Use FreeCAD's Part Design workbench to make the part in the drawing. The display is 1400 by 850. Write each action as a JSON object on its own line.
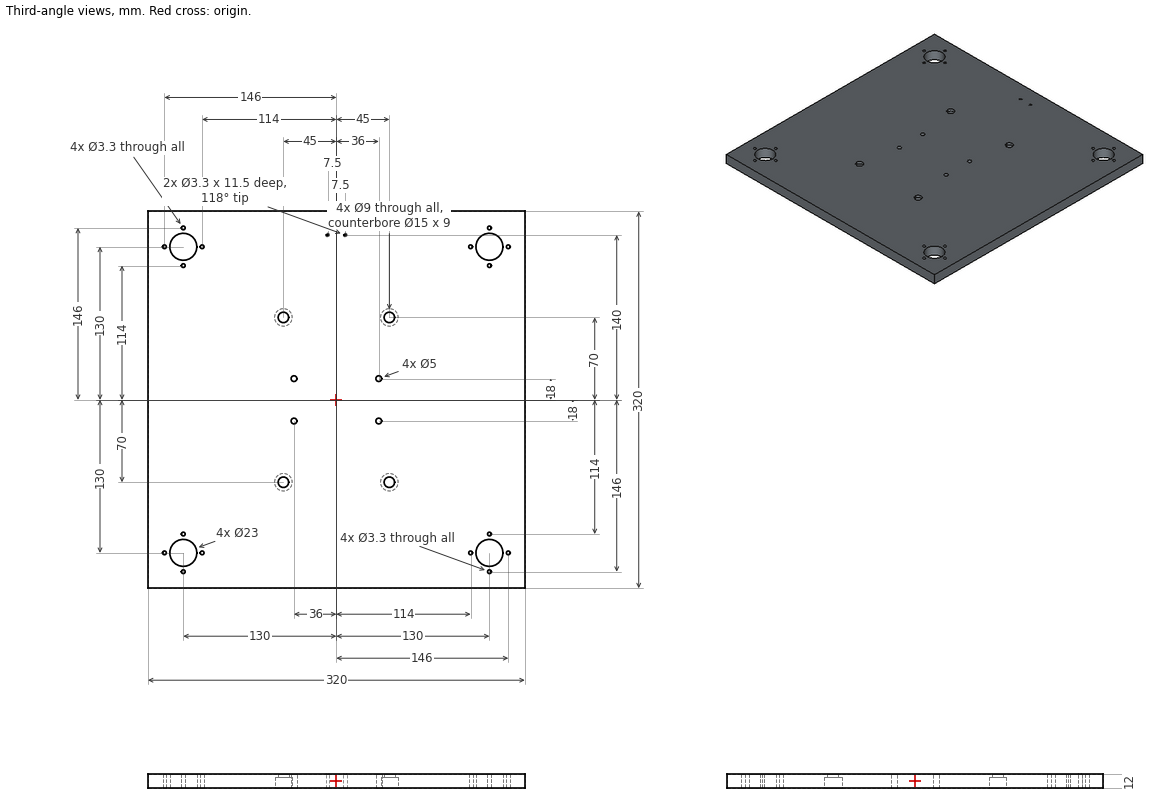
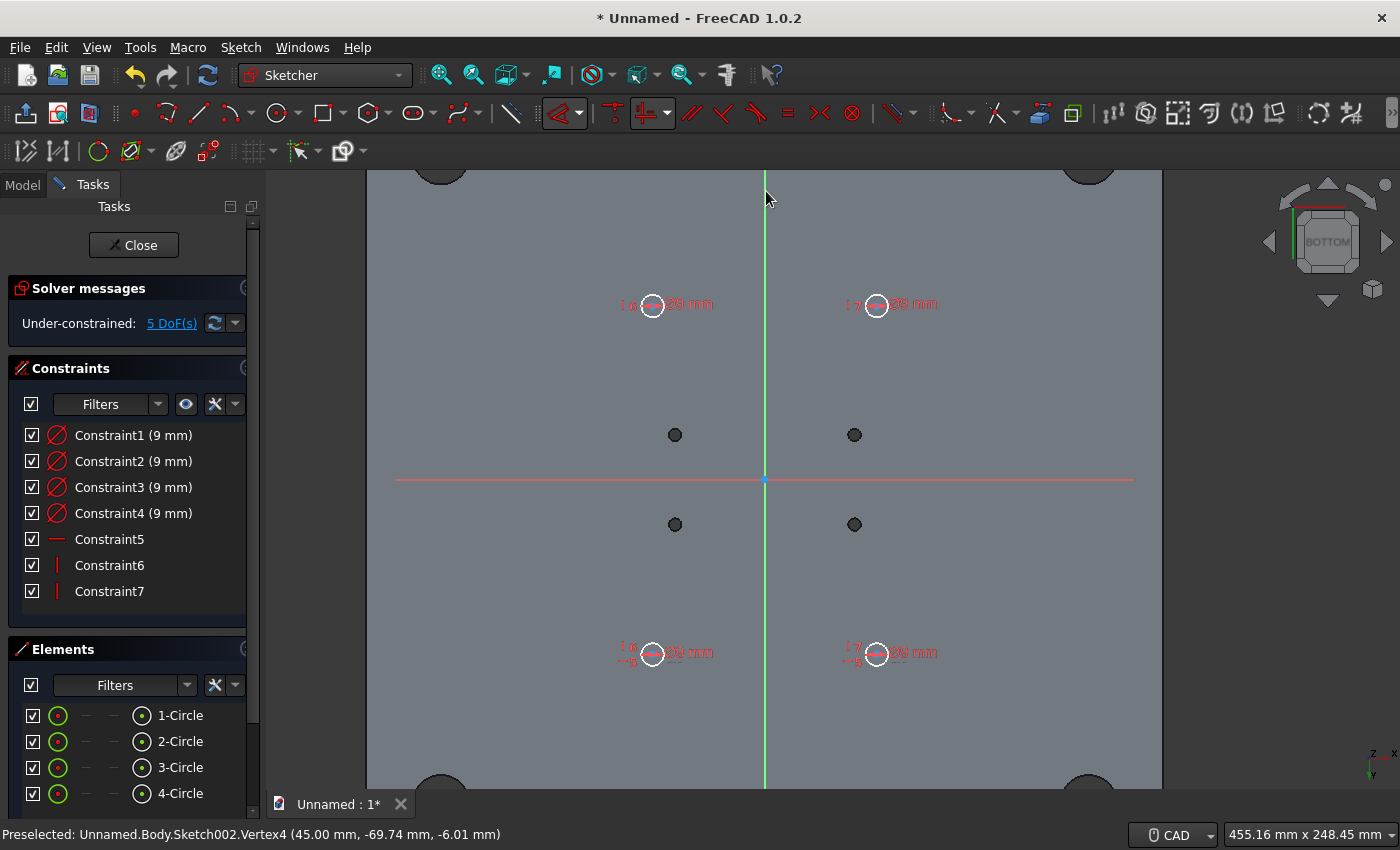
{"action": "left_click", "coordinate": [653, 306]}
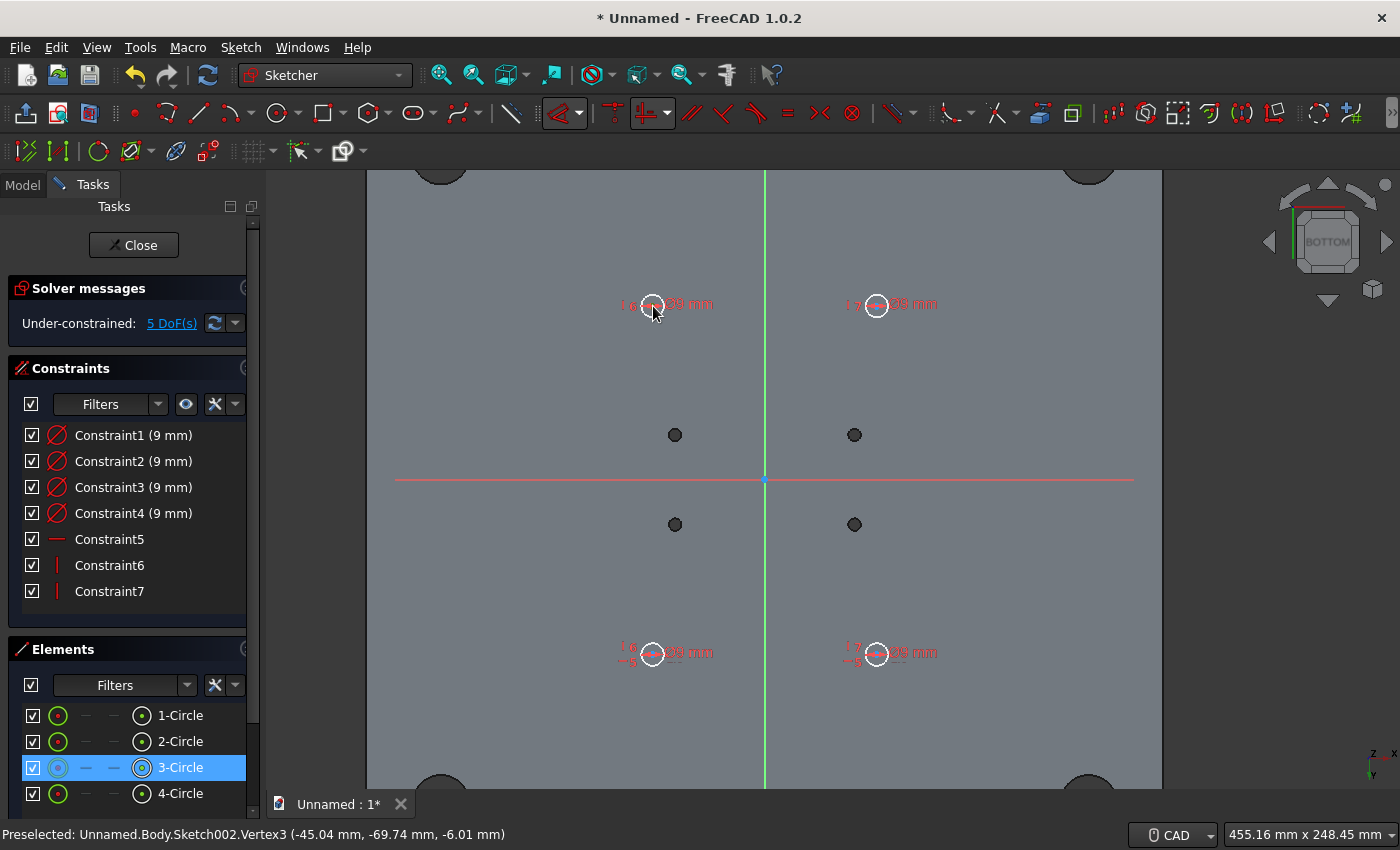
{"action": "left_click", "coordinate": [877, 306]}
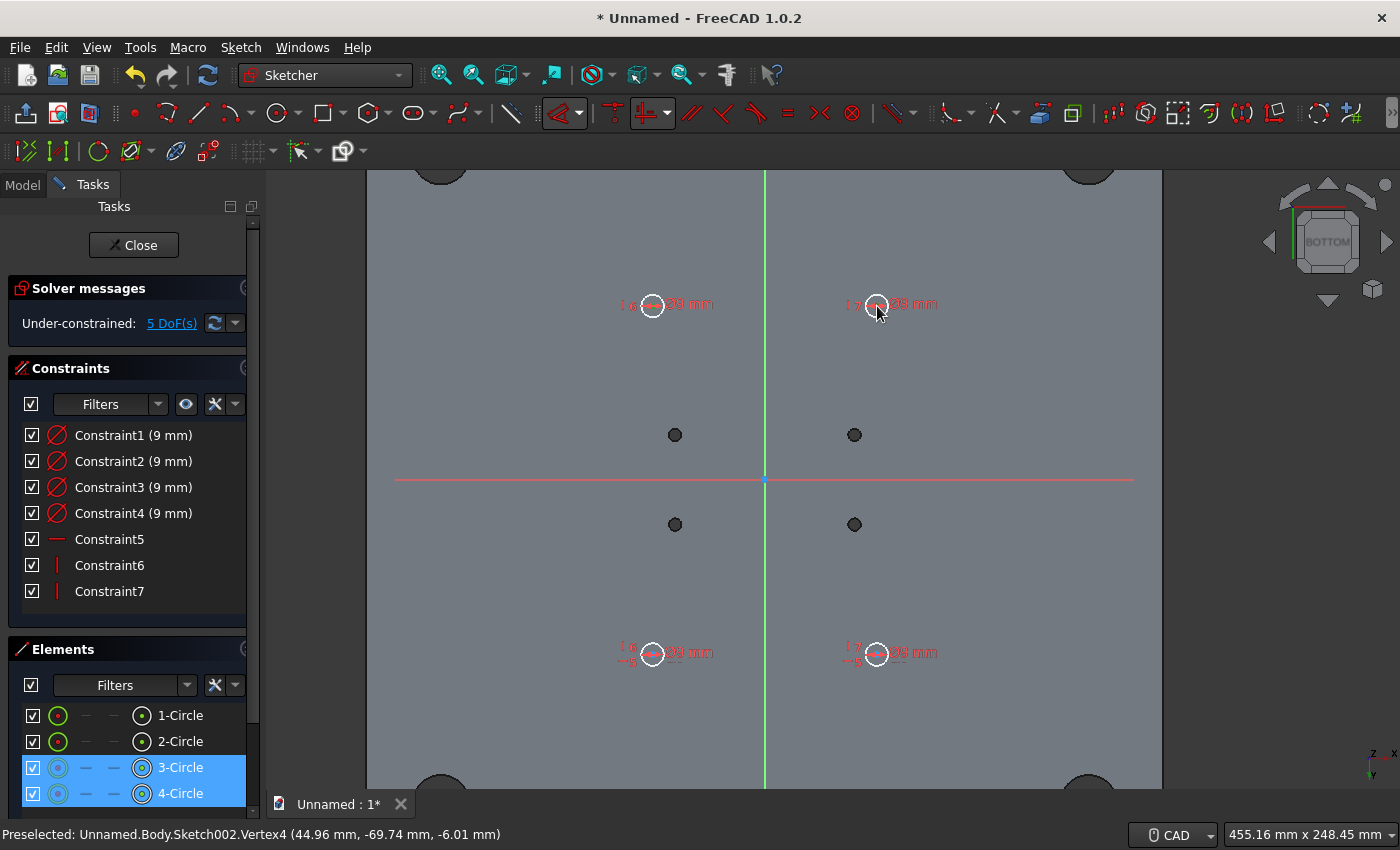
{"action": "left_click", "coordinate": [670, 114]}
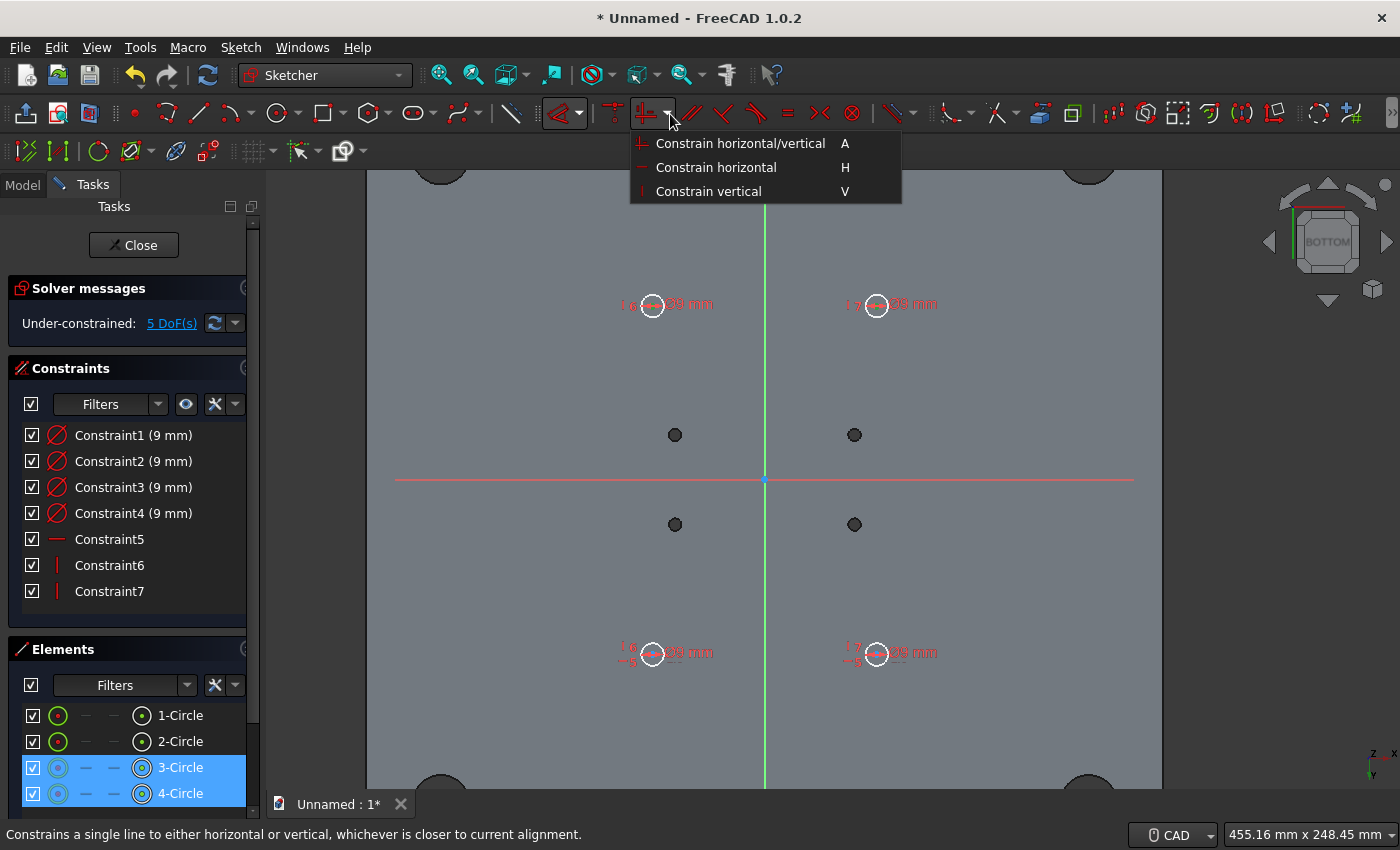
{"action": "left_click", "coordinate": [766, 167]}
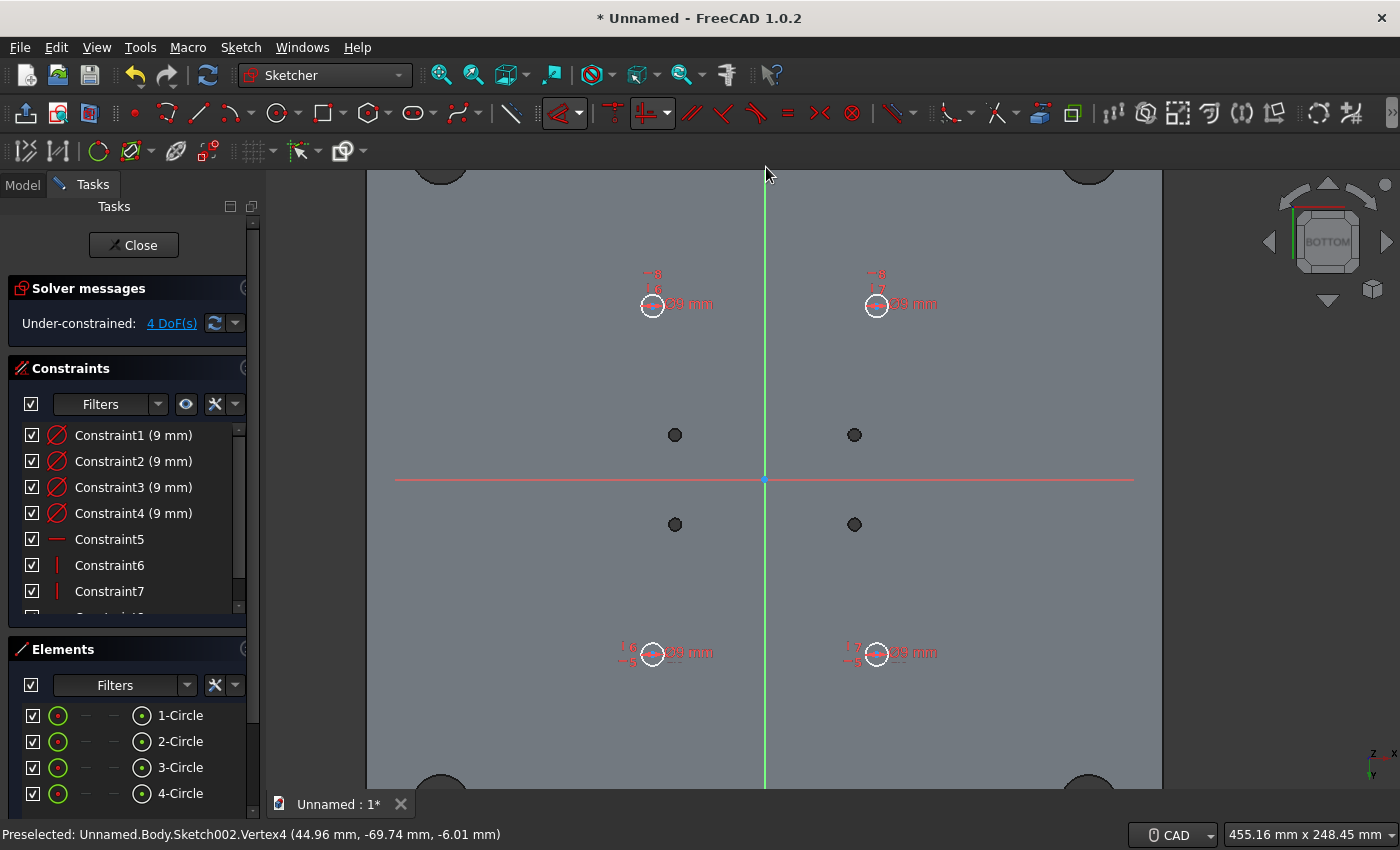
{"action": "left_click", "coordinate": [877, 655]}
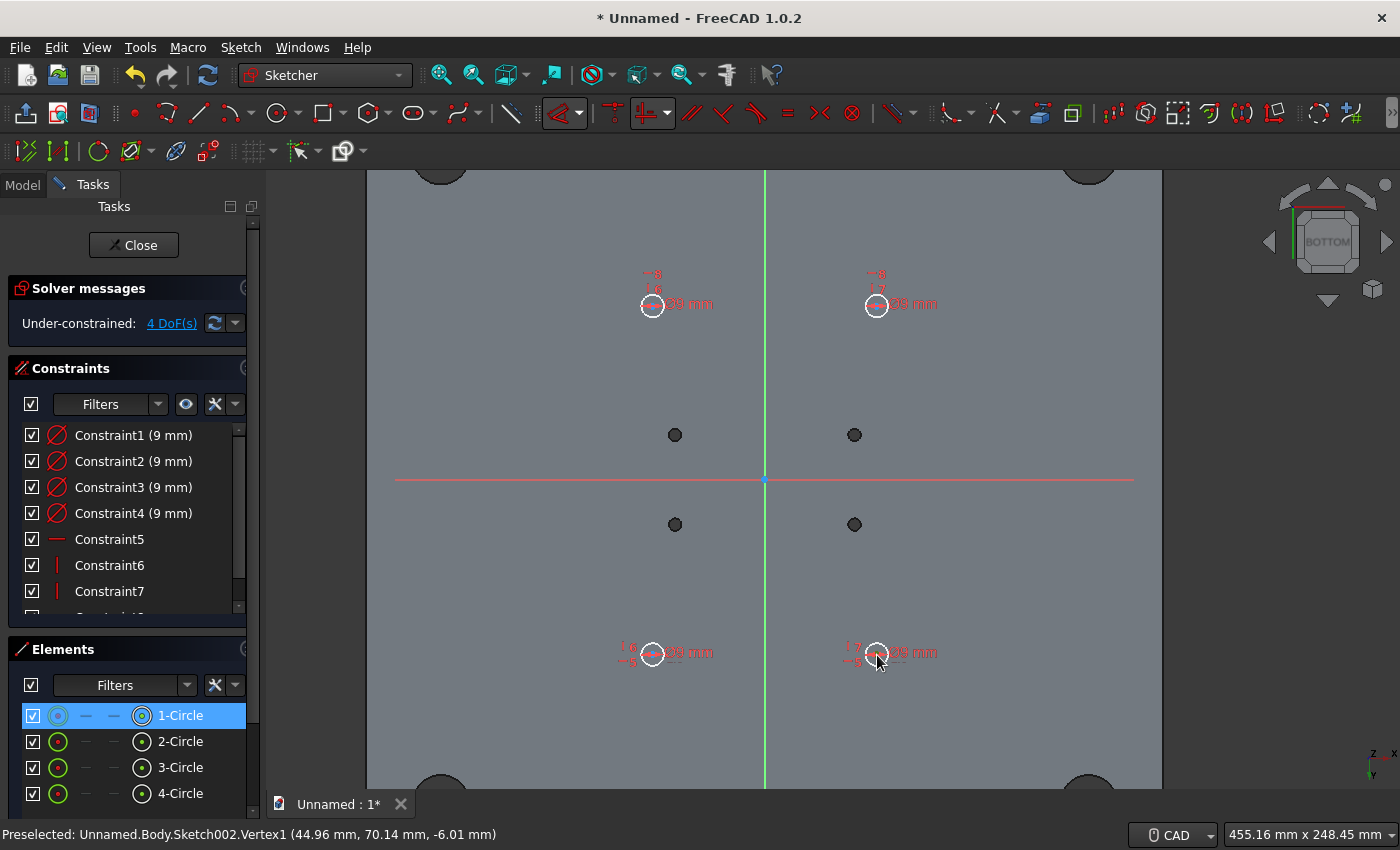
{"action": "left_click", "coordinate": [582, 114]}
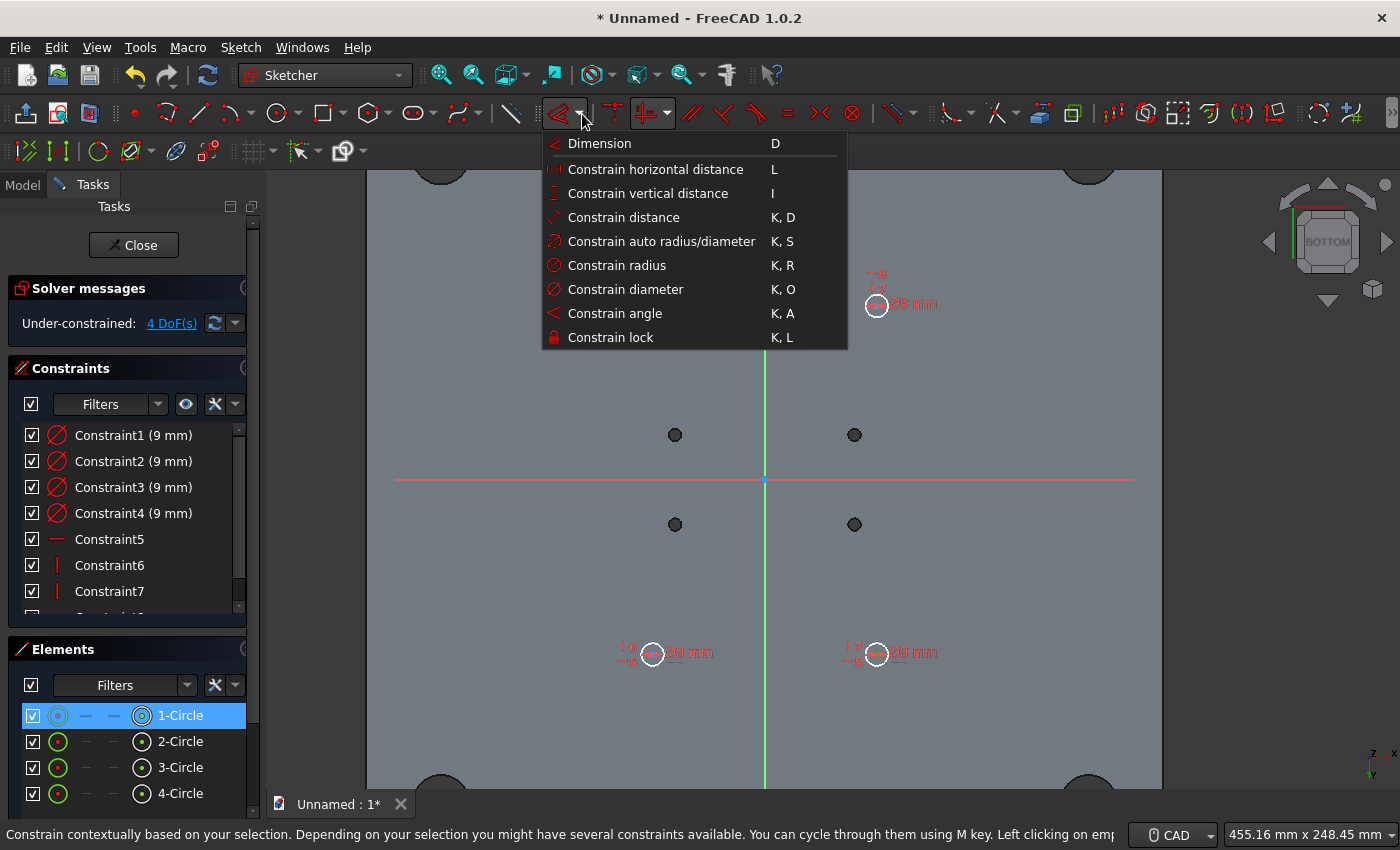
{"action": "left_click", "coordinate": [695, 169]}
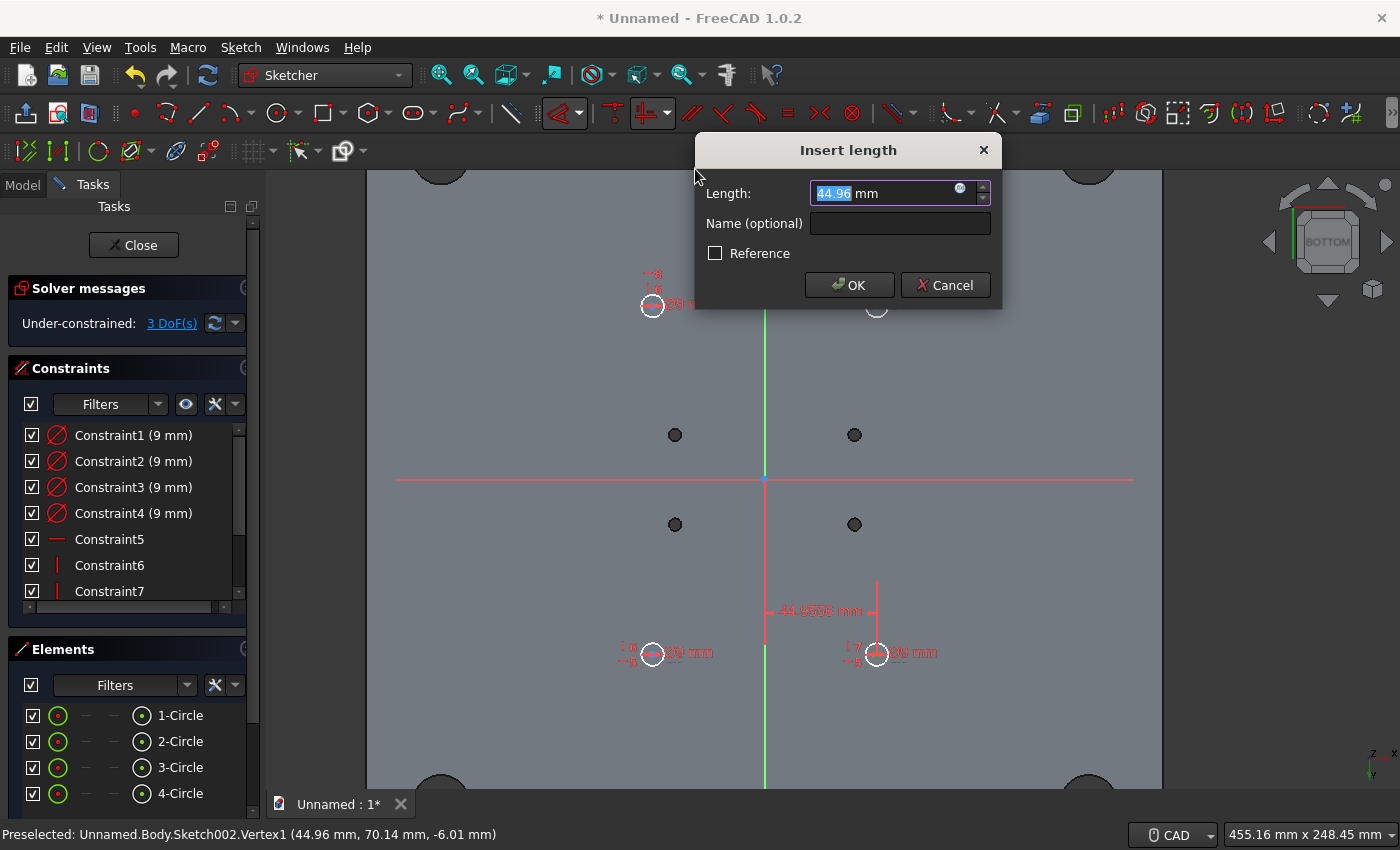
{"action": "type", "text": "45"}
{"action": "key", "text": "Return"}